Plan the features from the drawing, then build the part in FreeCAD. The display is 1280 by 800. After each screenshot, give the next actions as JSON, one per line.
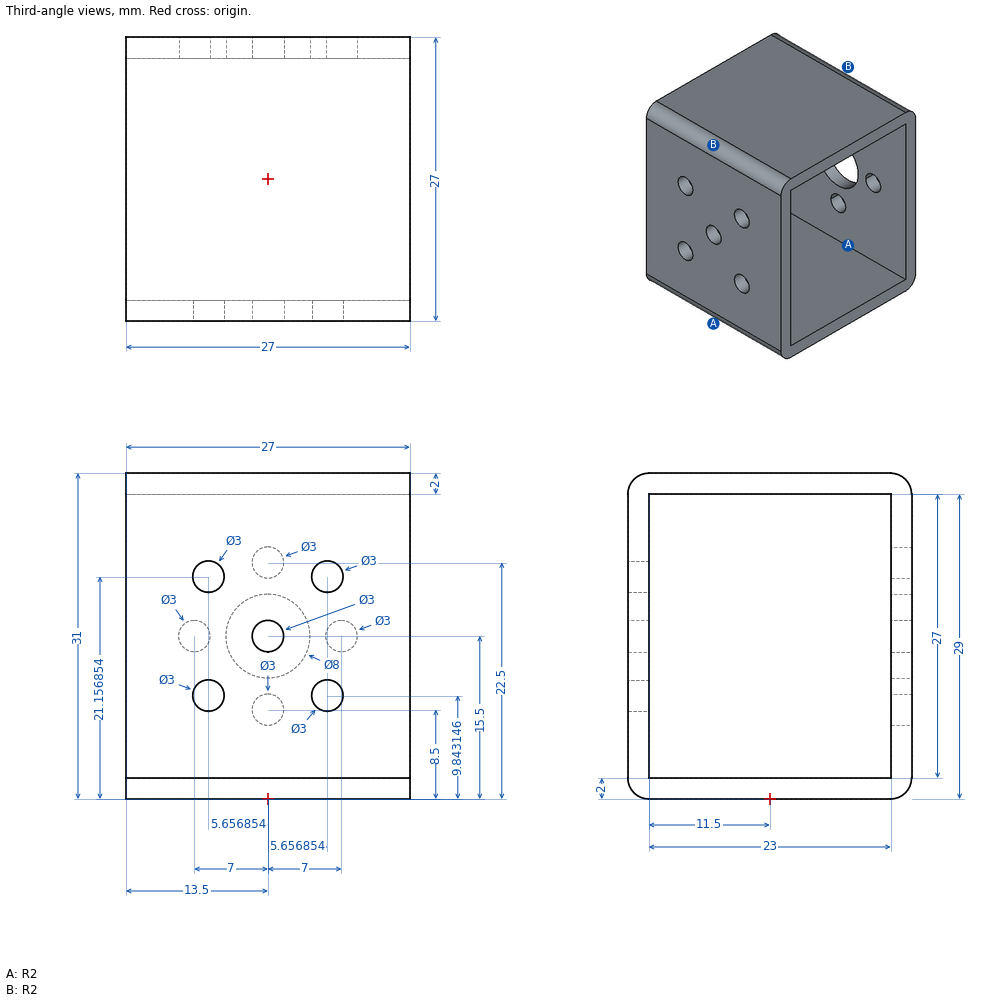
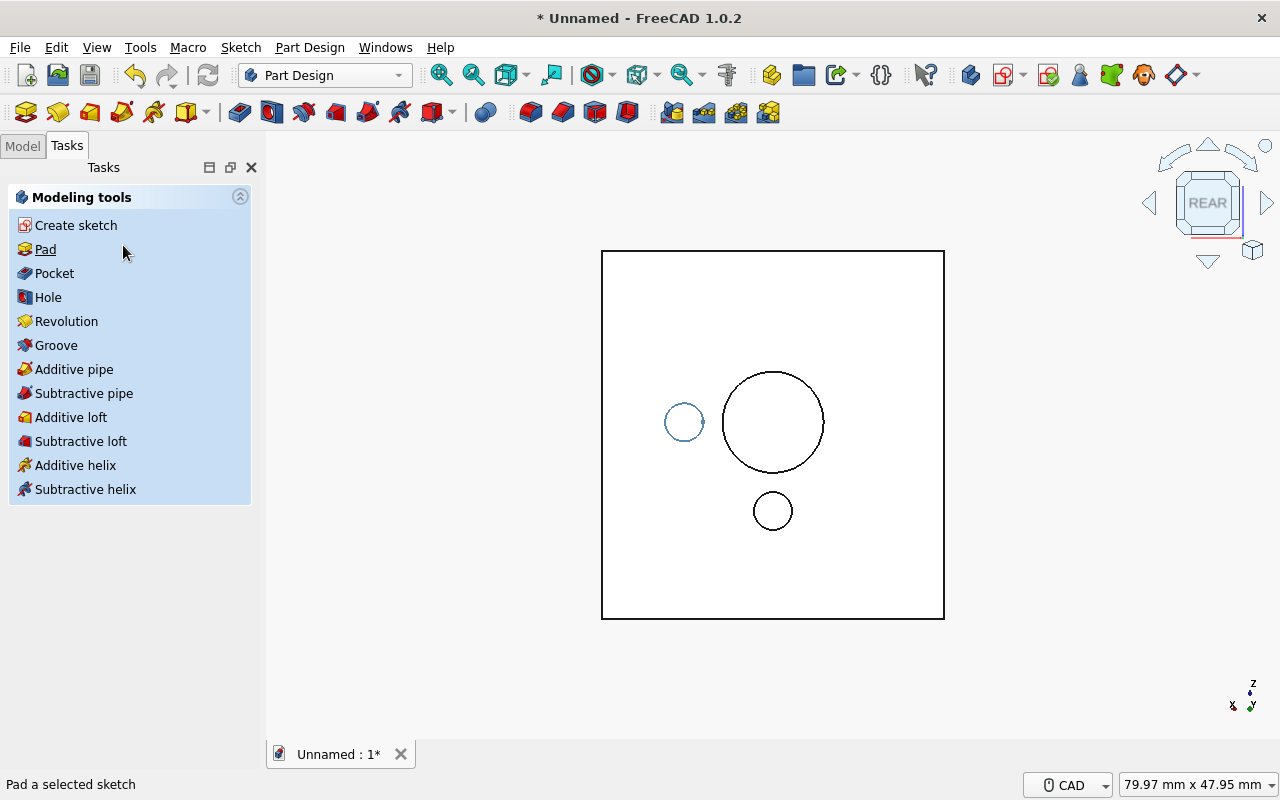
{"action": "left_click", "coordinate": [240, 112]}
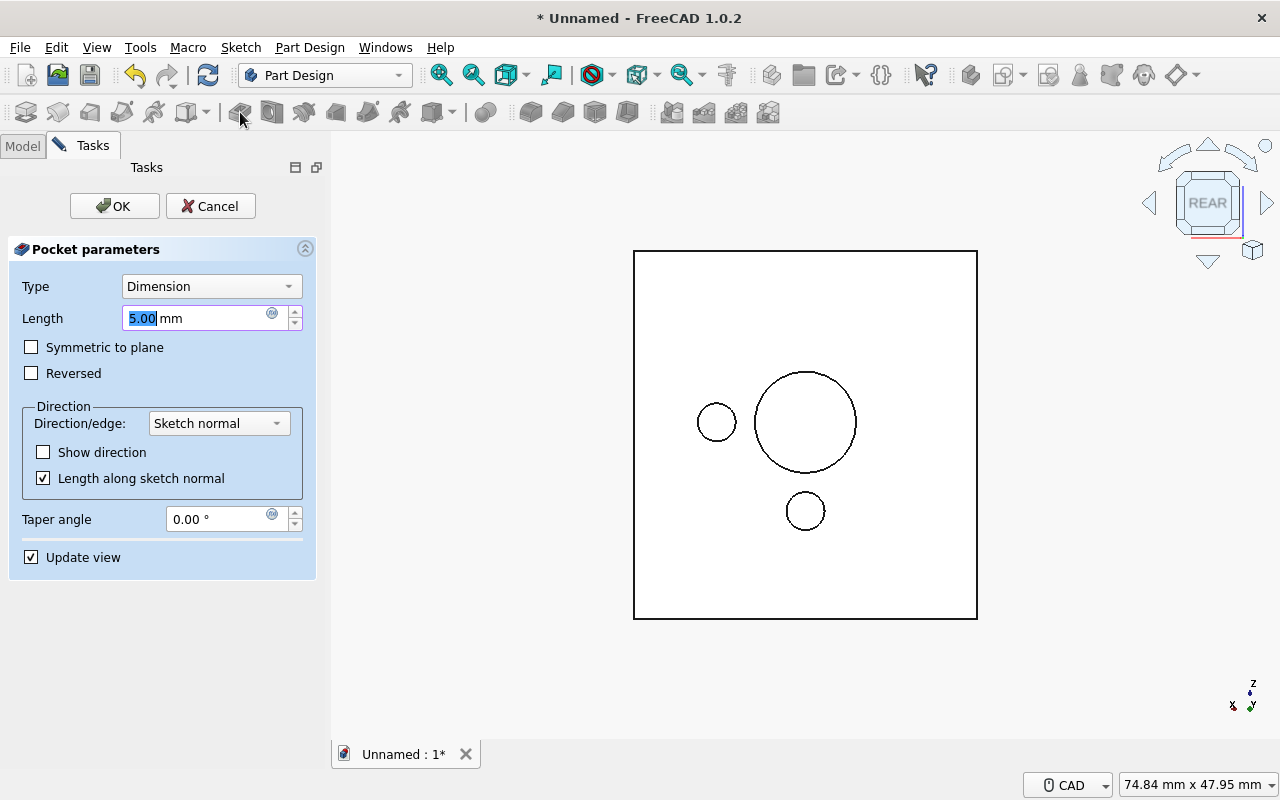
{"action": "left_click", "coordinate": [212, 286]}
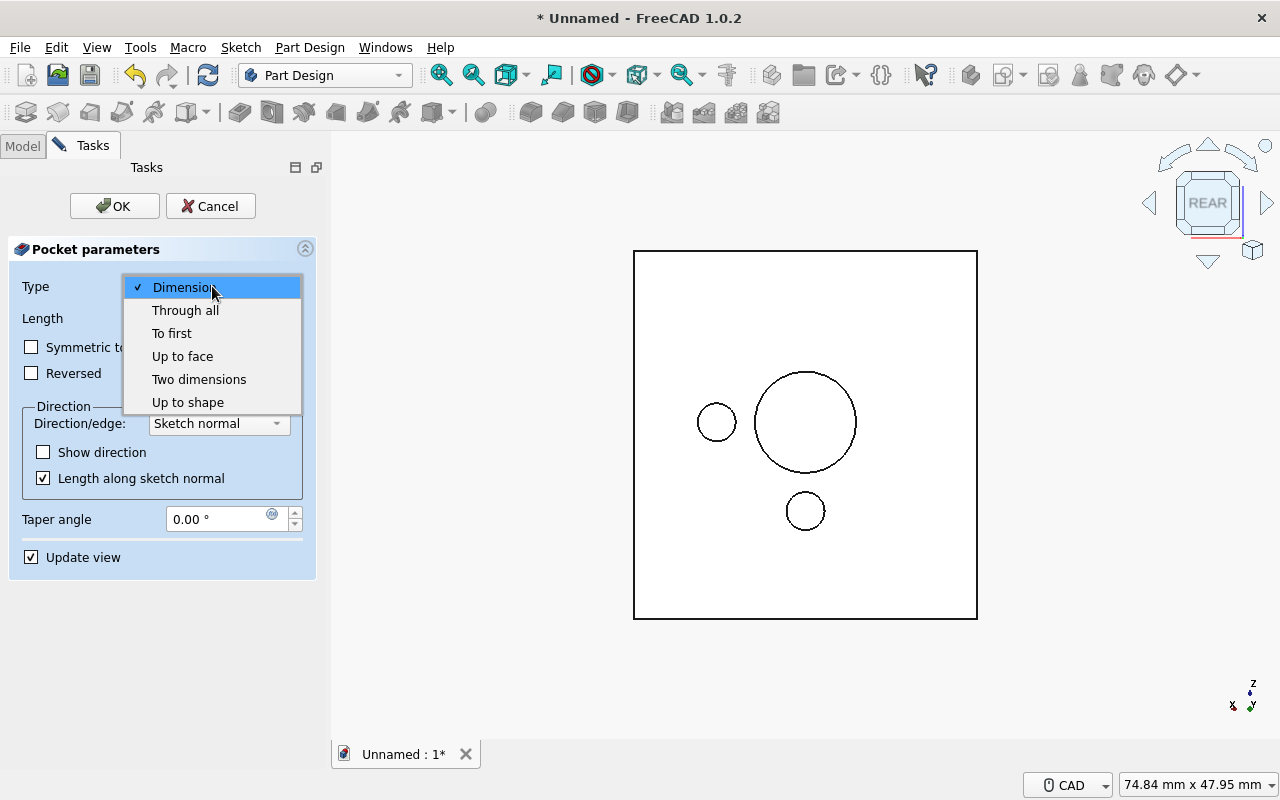
{"action": "left_click", "coordinate": [212, 334]}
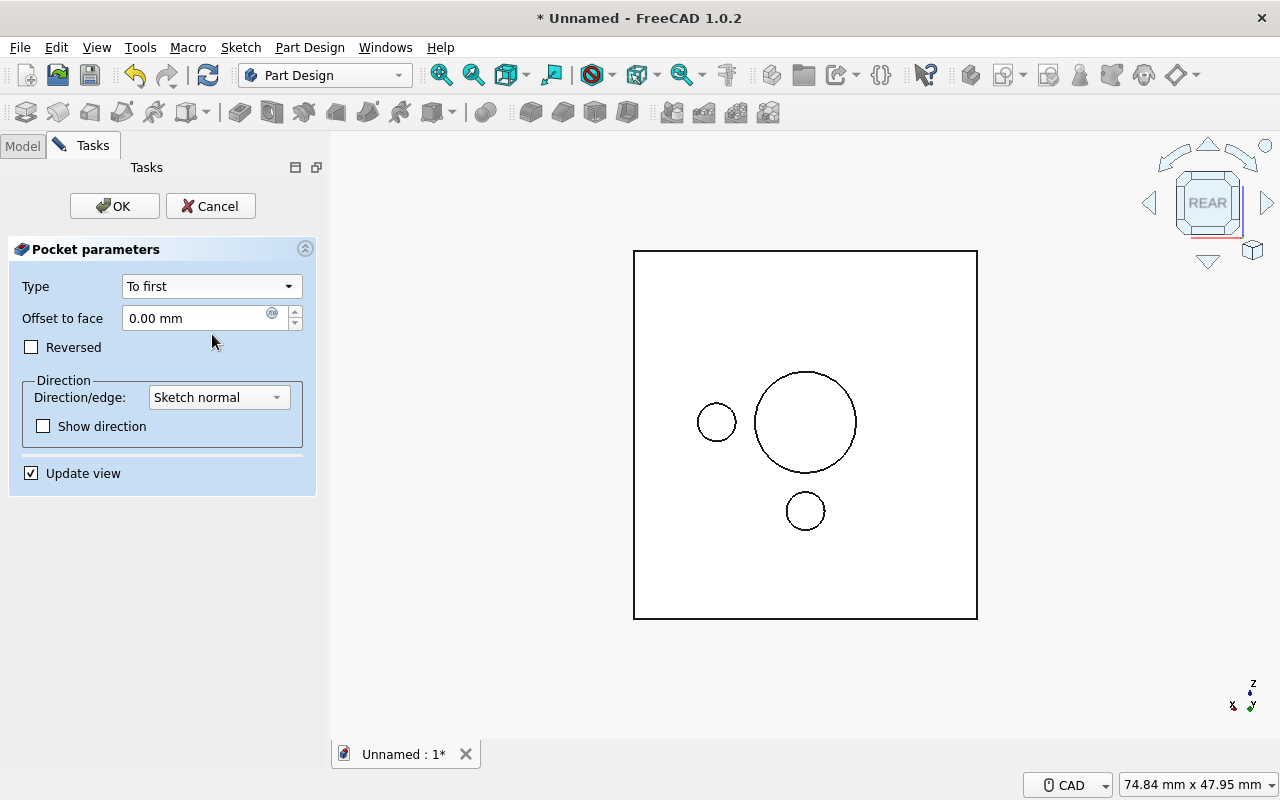
{"action": "left_click", "coordinate": [115, 206]}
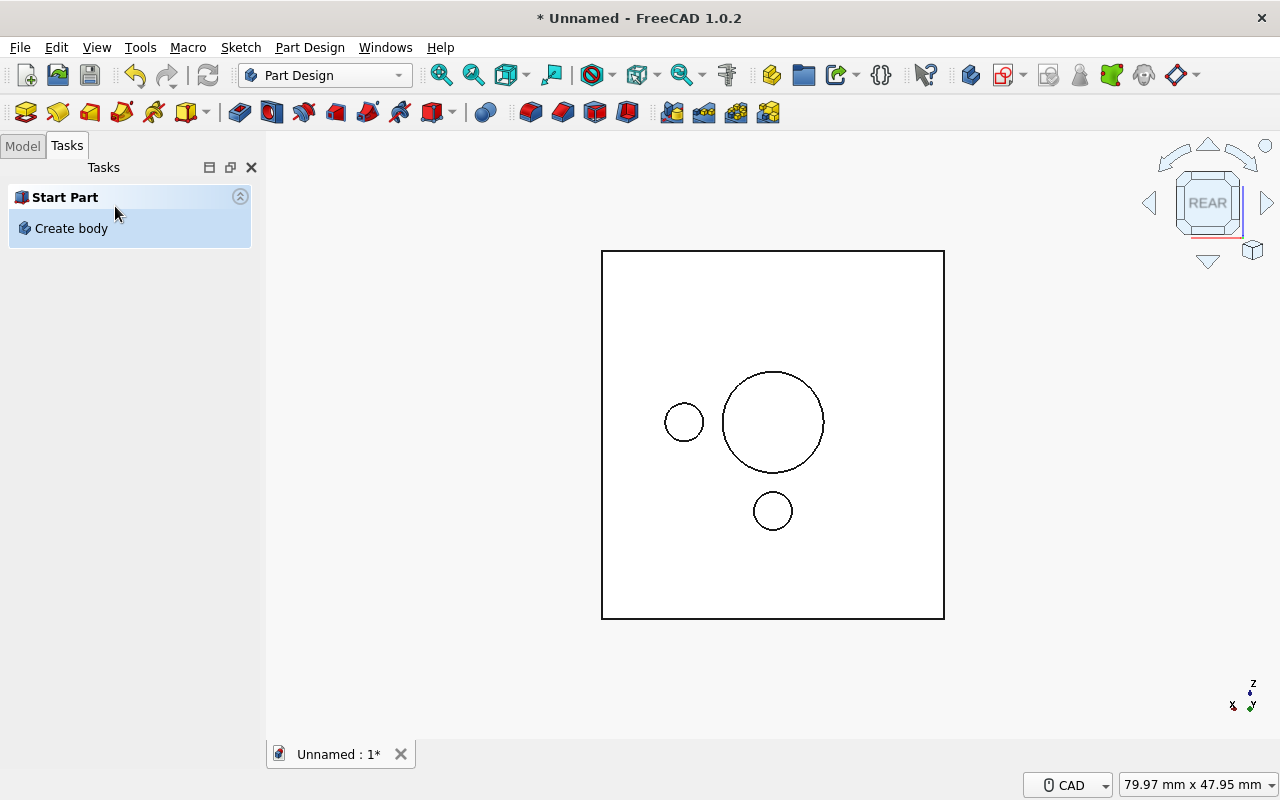
{"action": "left_click", "coordinate": [675, 329]}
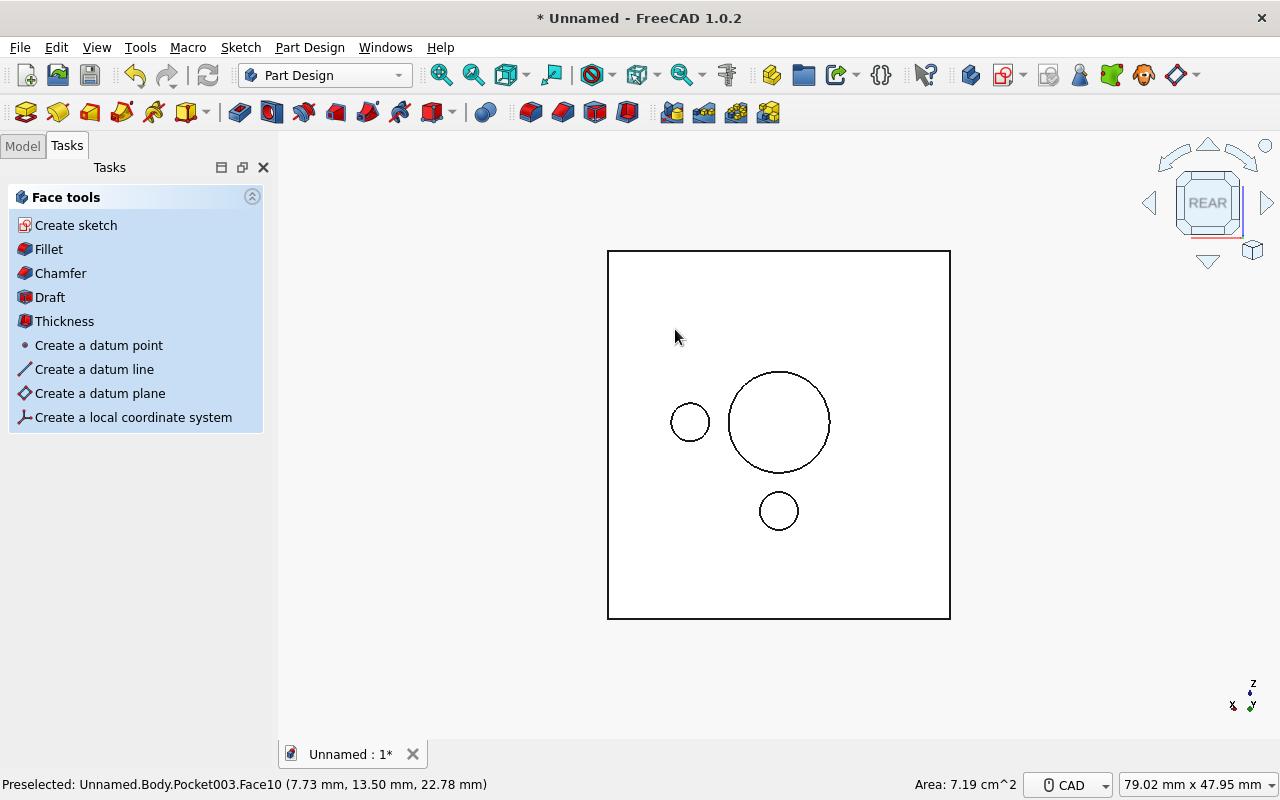
{"action": "left_click", "coordinate": [1004, 76]}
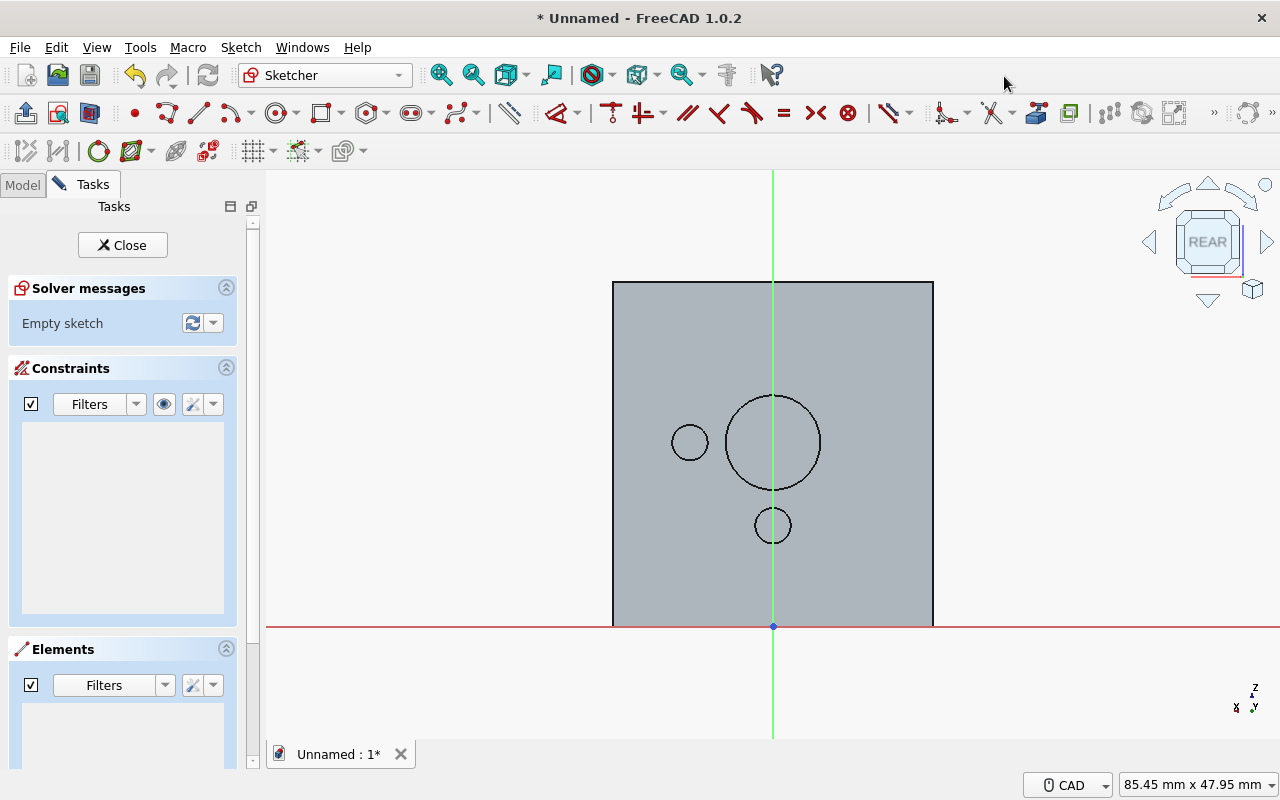
{"action": "scroll", "coordinate": [780, 350], "scroll_direction": "up", "scroll_amount": 12}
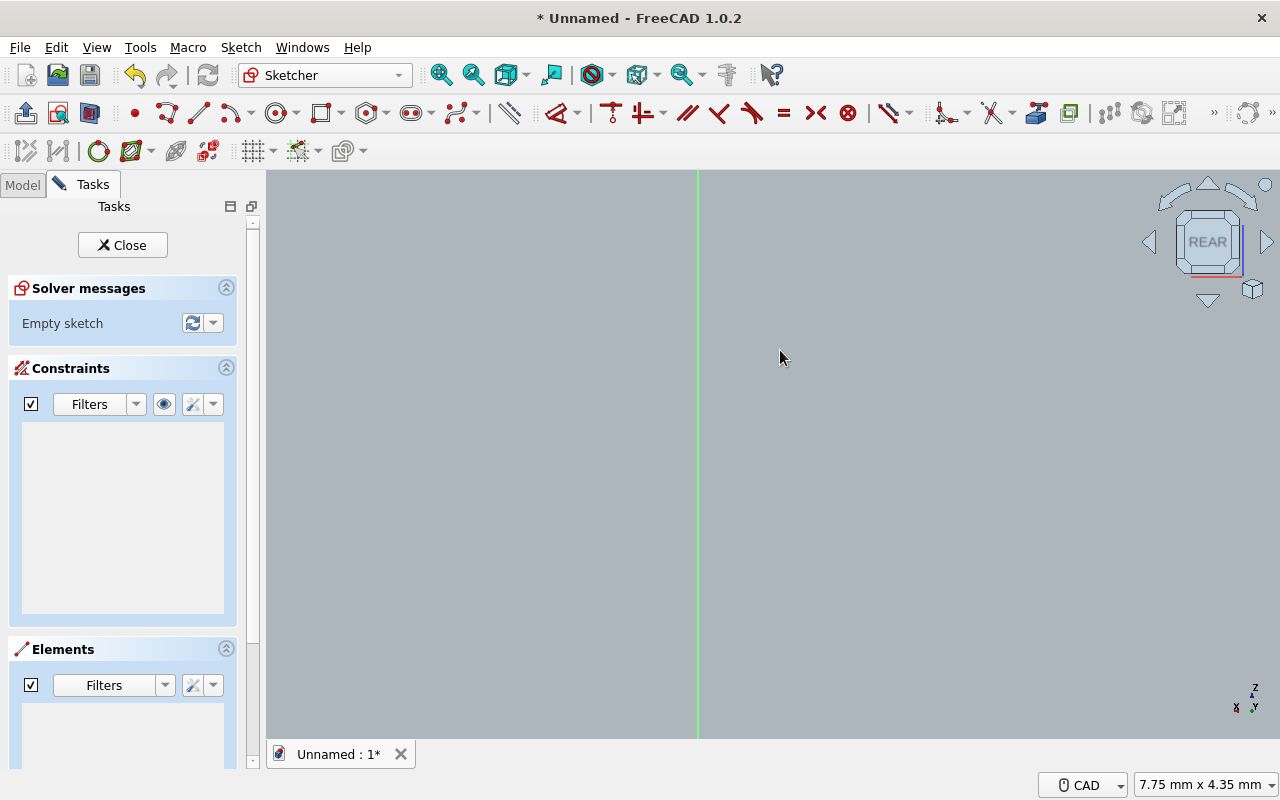
{"action": "left_click", "coordinate": [276, 114]}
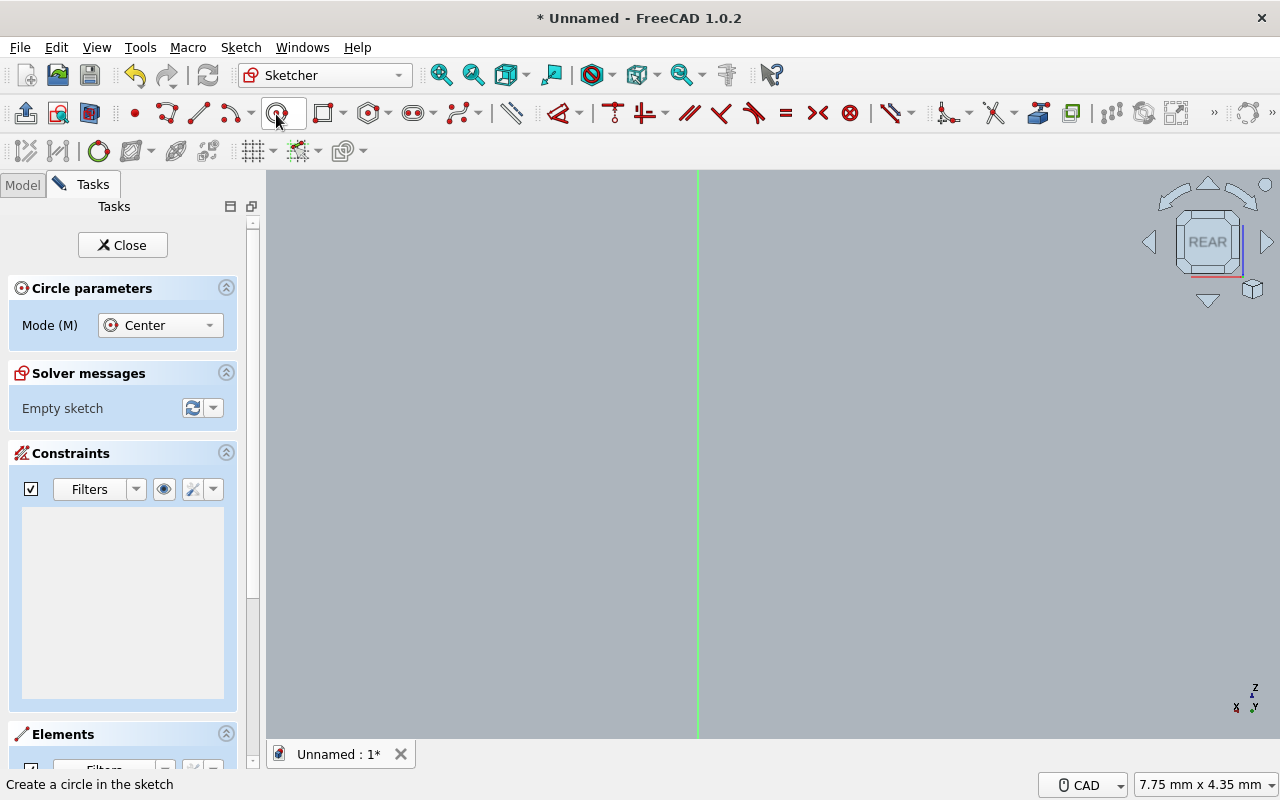
{"action": "left_click", "coordinate": [698, 452]}
{"action": "mouse_move", "coordinate": [837, 313]}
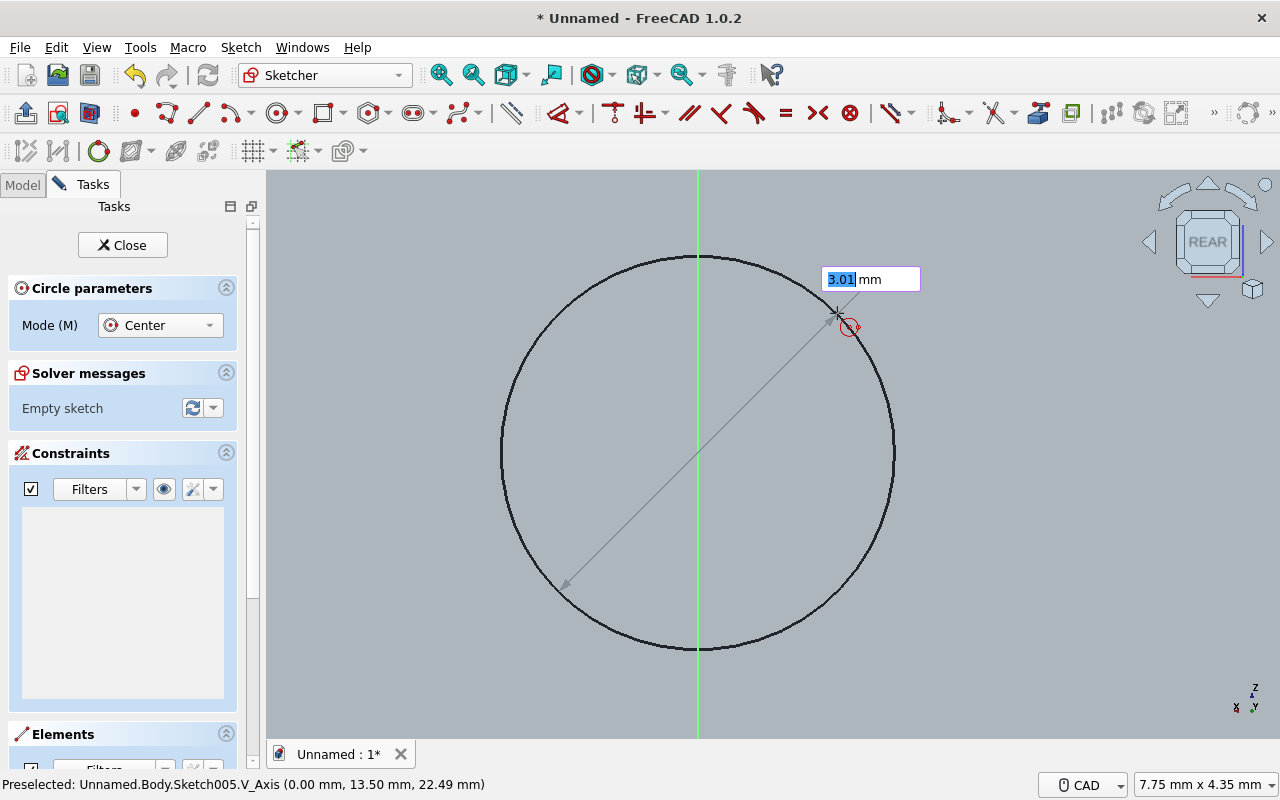
{"action": "type", "text": "3"}
{"action": "key", "text": "Return"}
{"action": "key", "text": "Escape"}